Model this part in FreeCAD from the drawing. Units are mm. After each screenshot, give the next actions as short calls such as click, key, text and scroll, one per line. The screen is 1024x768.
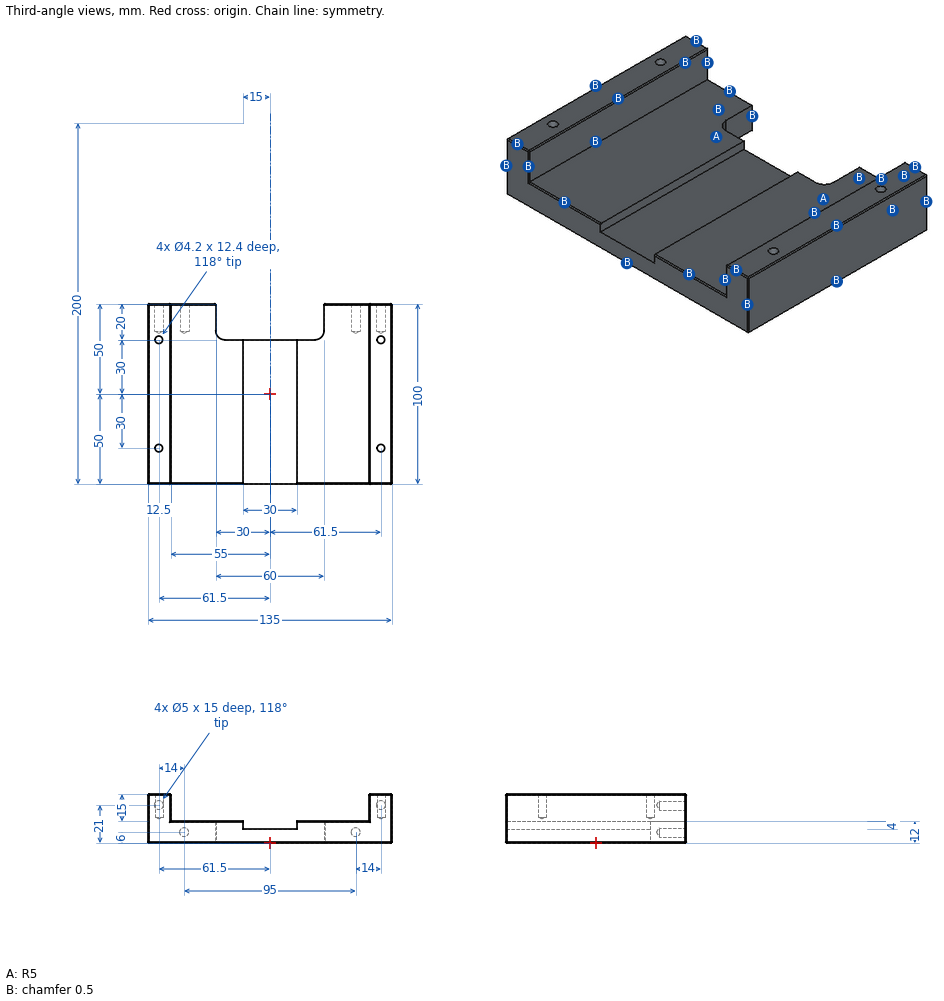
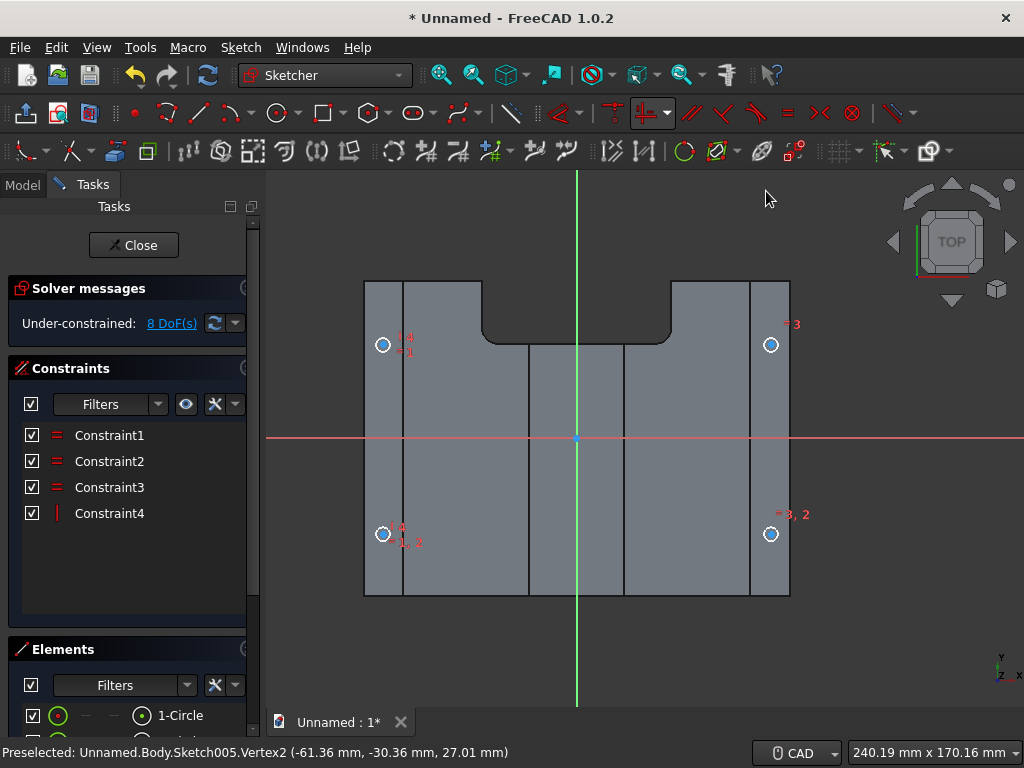
click(383, 534)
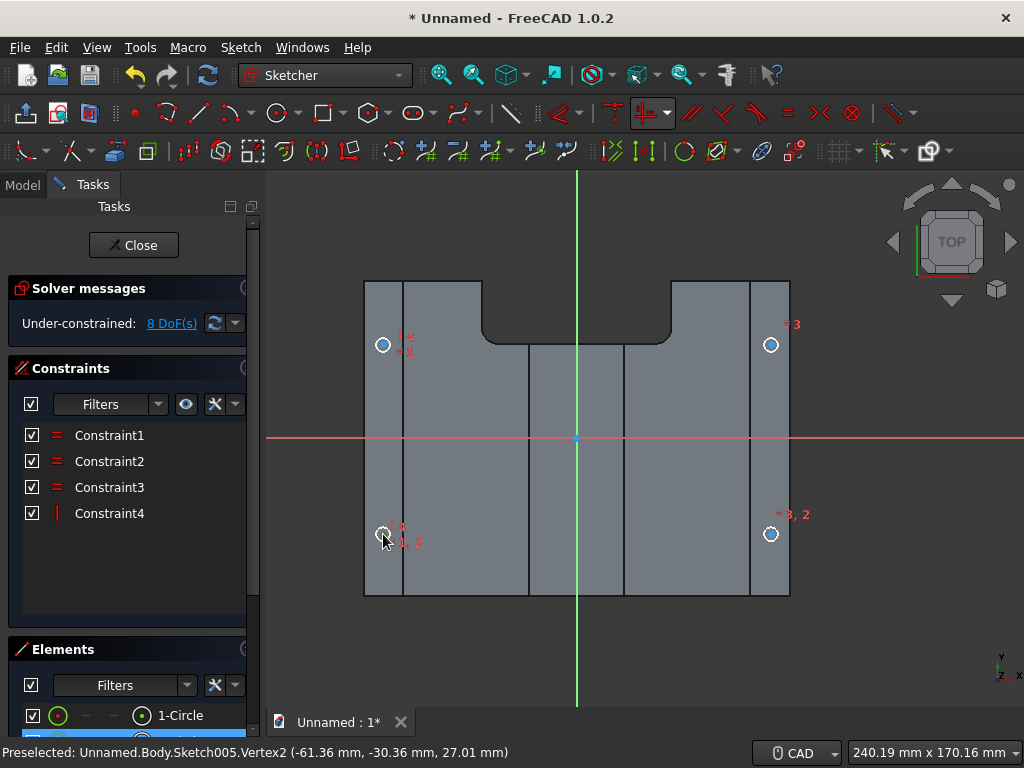
click(771, 534)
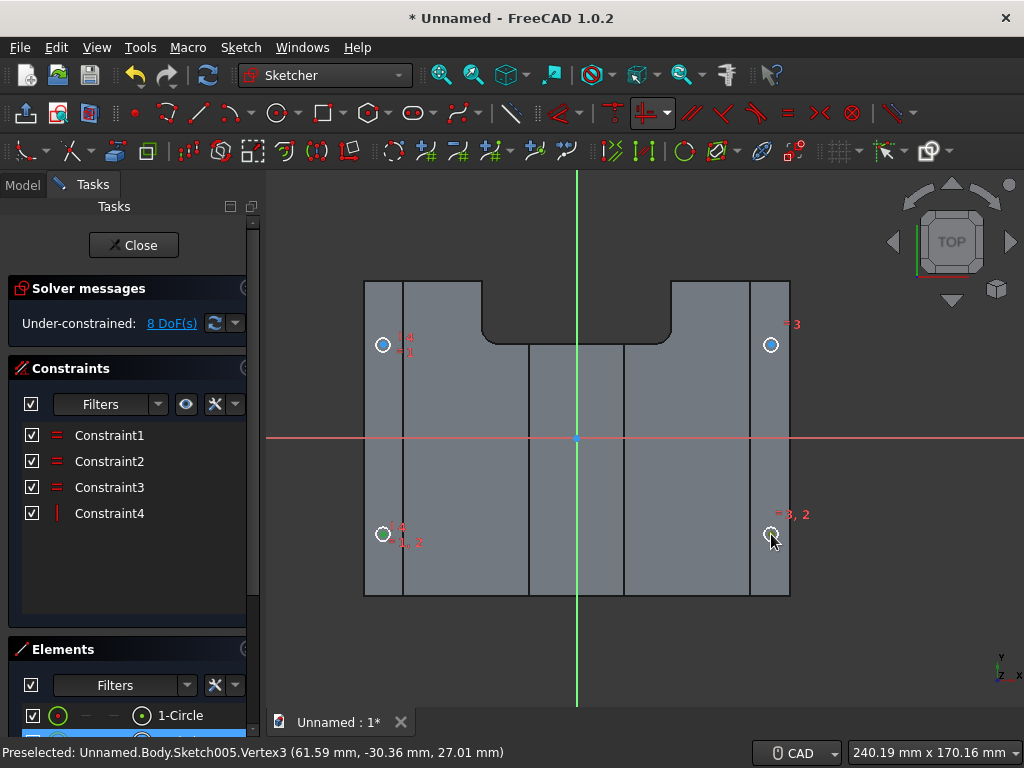
click(670, 114)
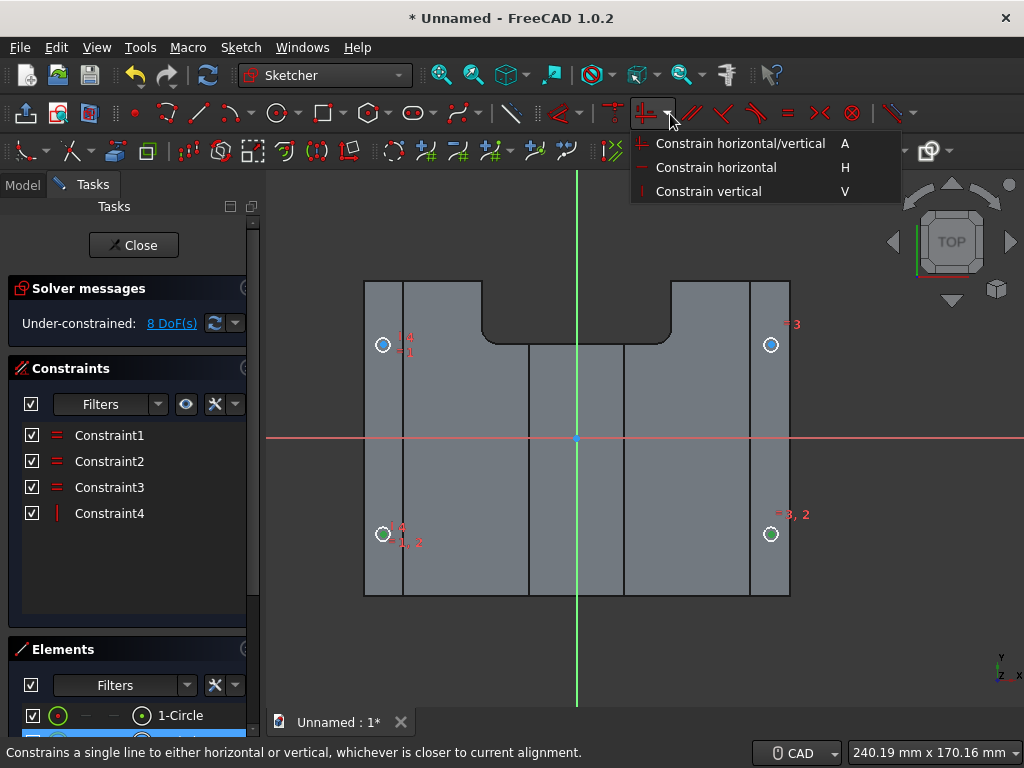
click(766, 167)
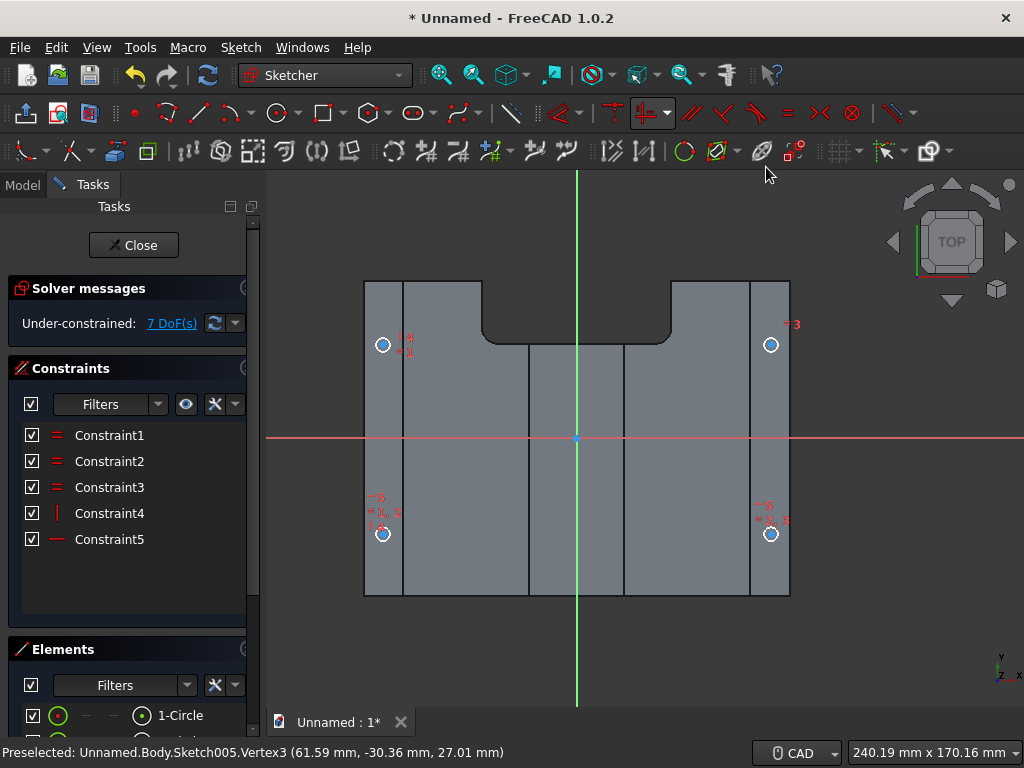
click(771, 534)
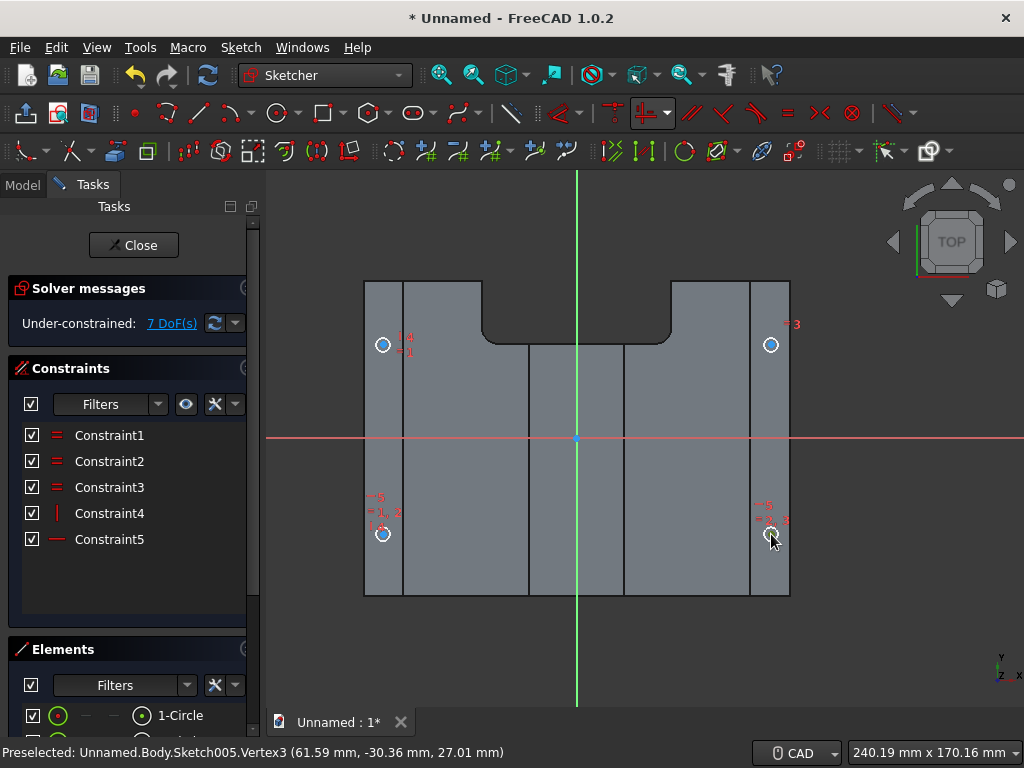
click(771, 345)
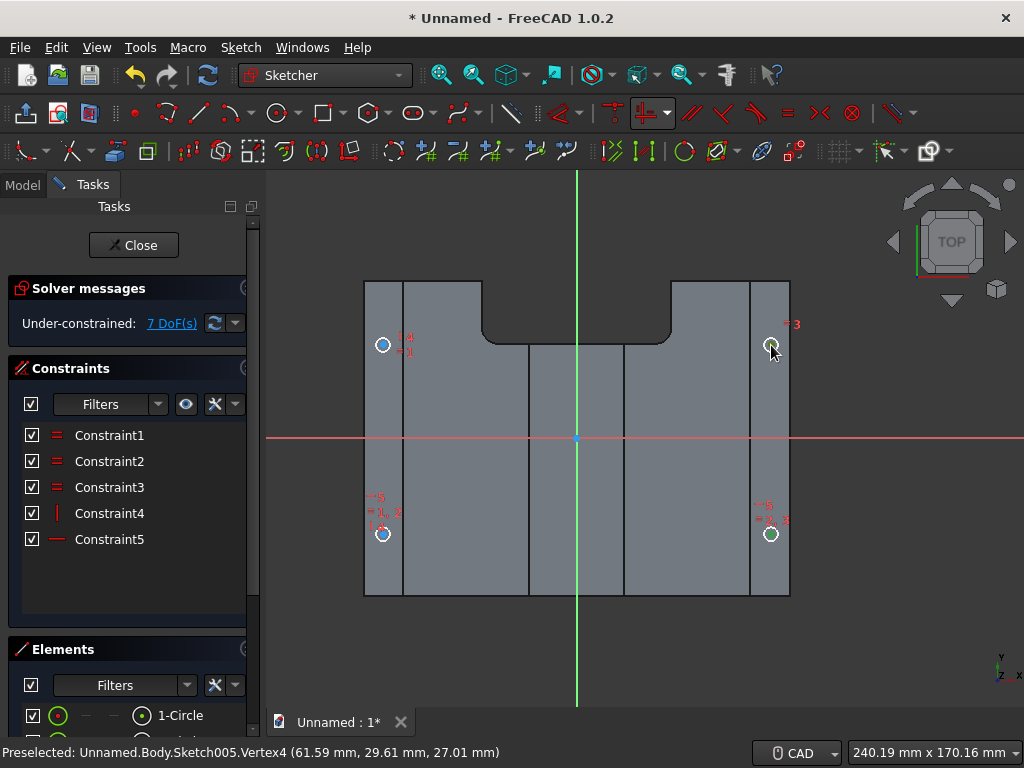
key(v)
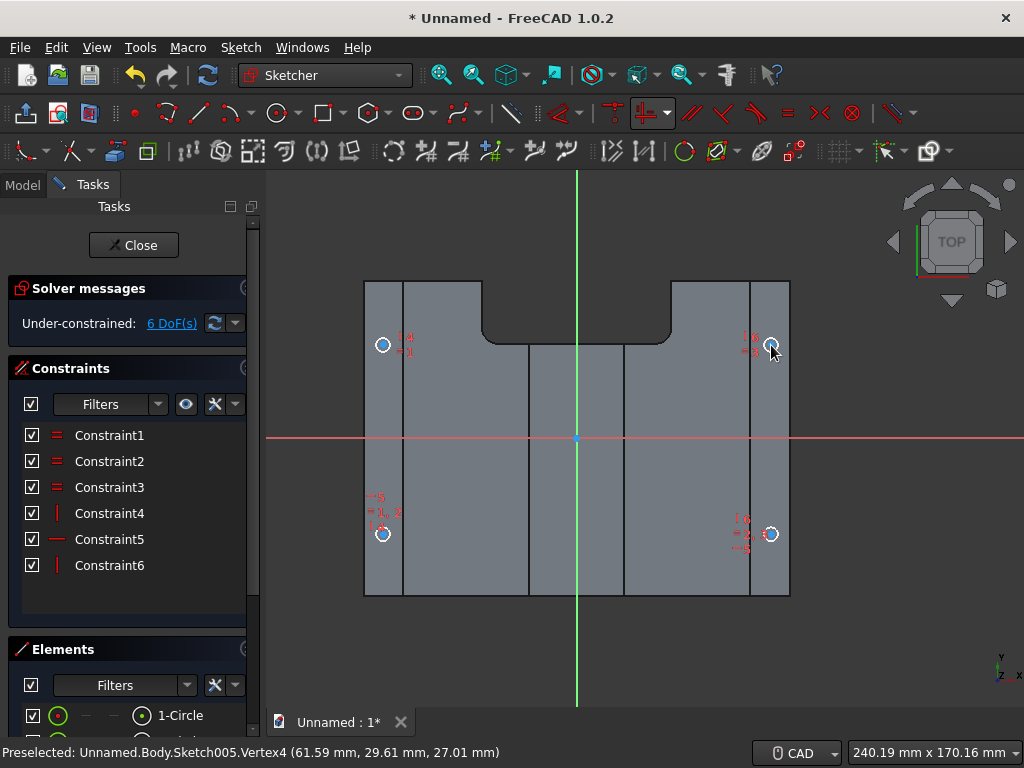
click(383, 345)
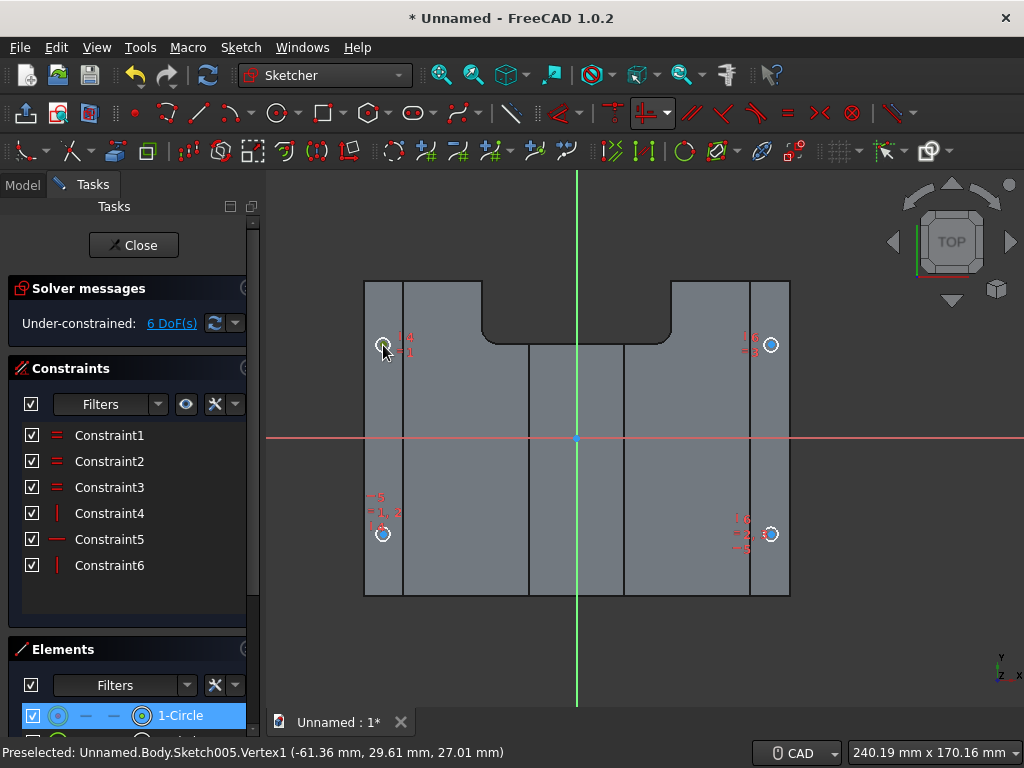
click(771, 345)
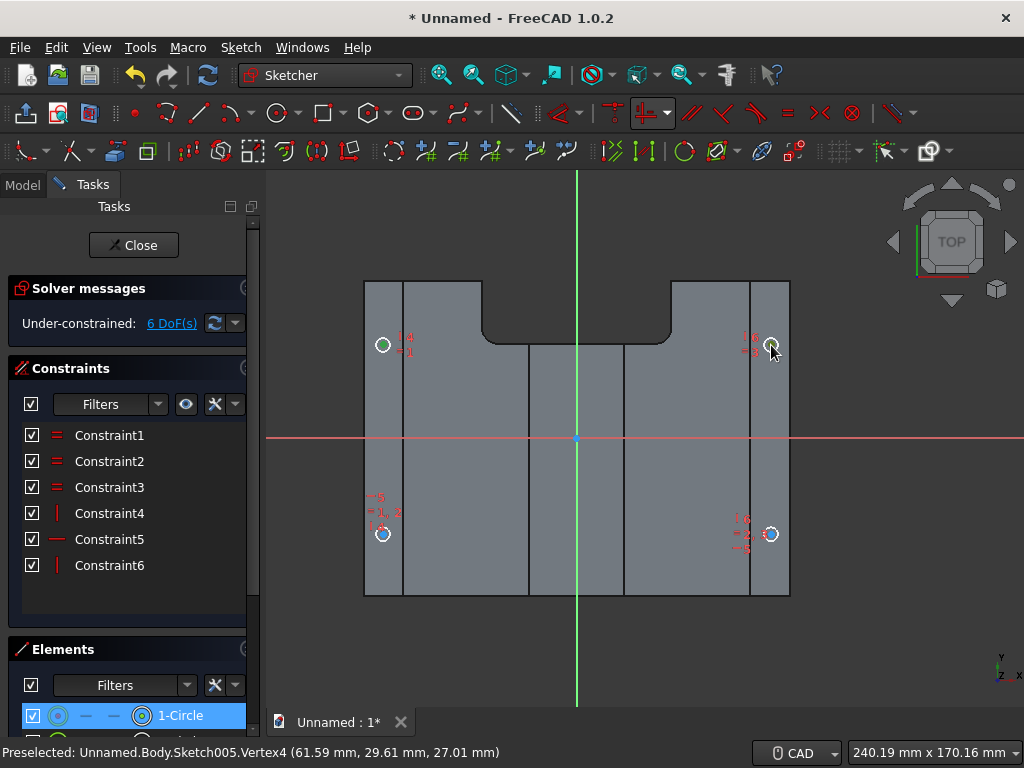
key(h)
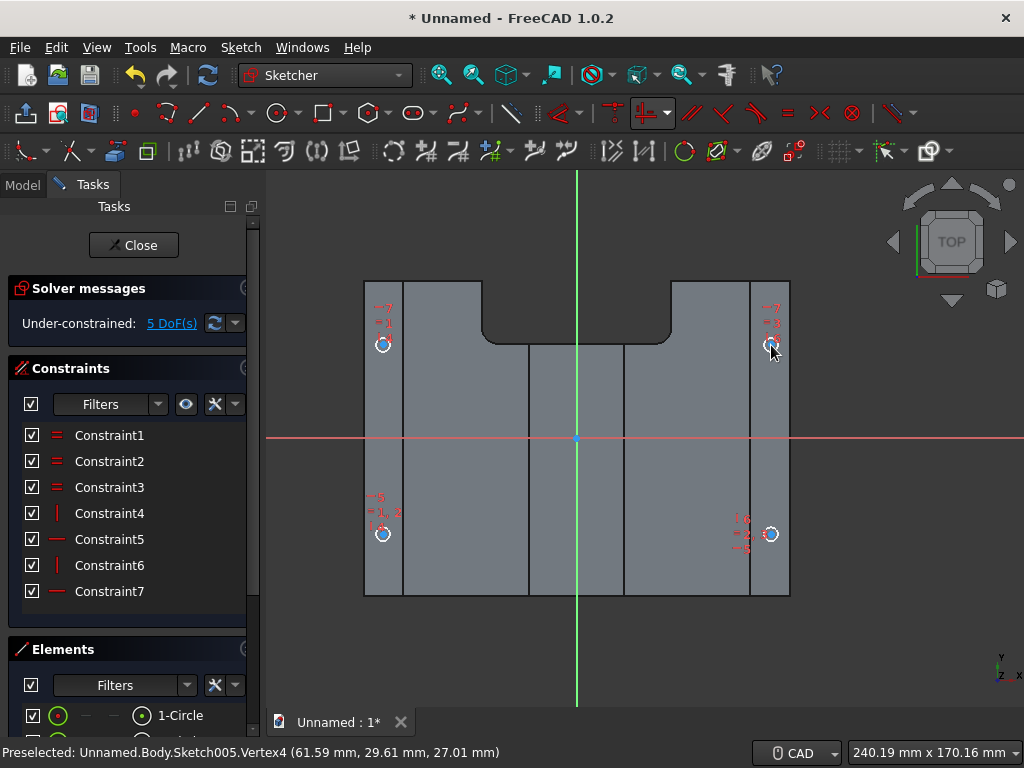
key(d)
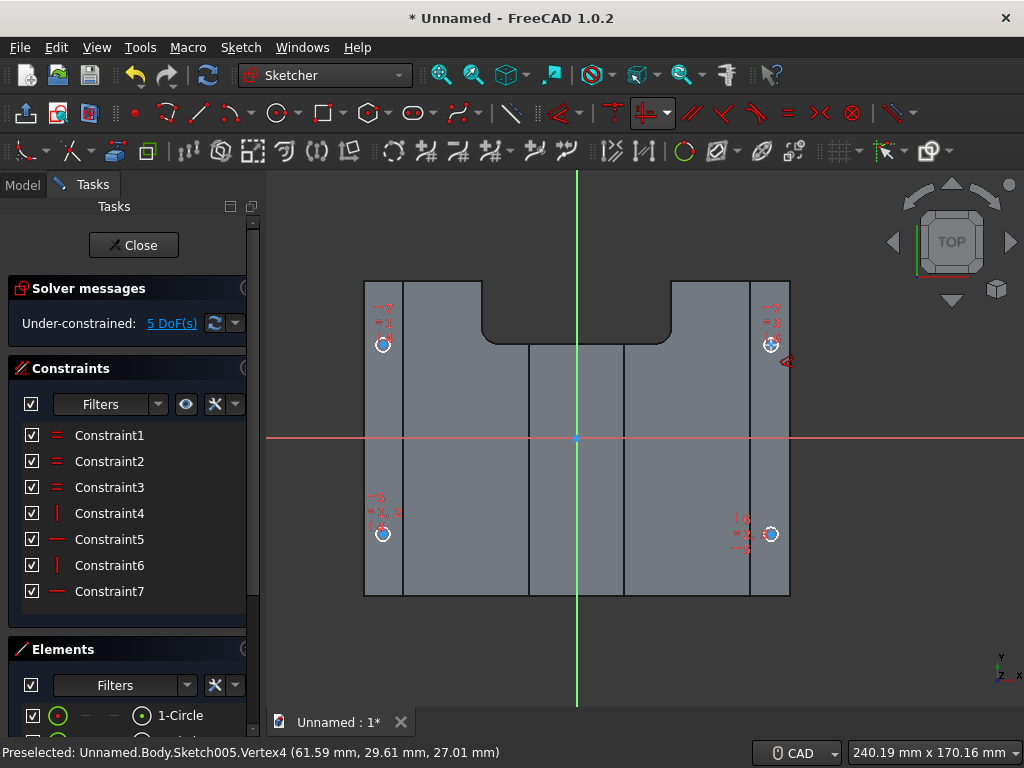
scroll(388, 340, up, 6)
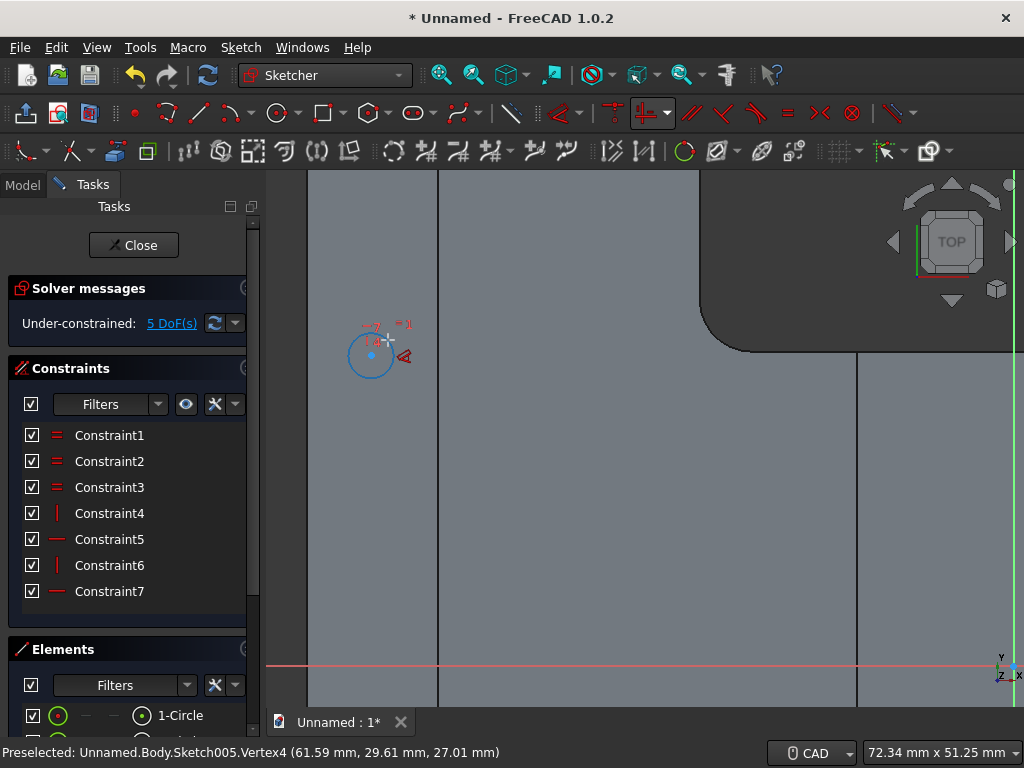
click(387, 340)
click(410, 317)